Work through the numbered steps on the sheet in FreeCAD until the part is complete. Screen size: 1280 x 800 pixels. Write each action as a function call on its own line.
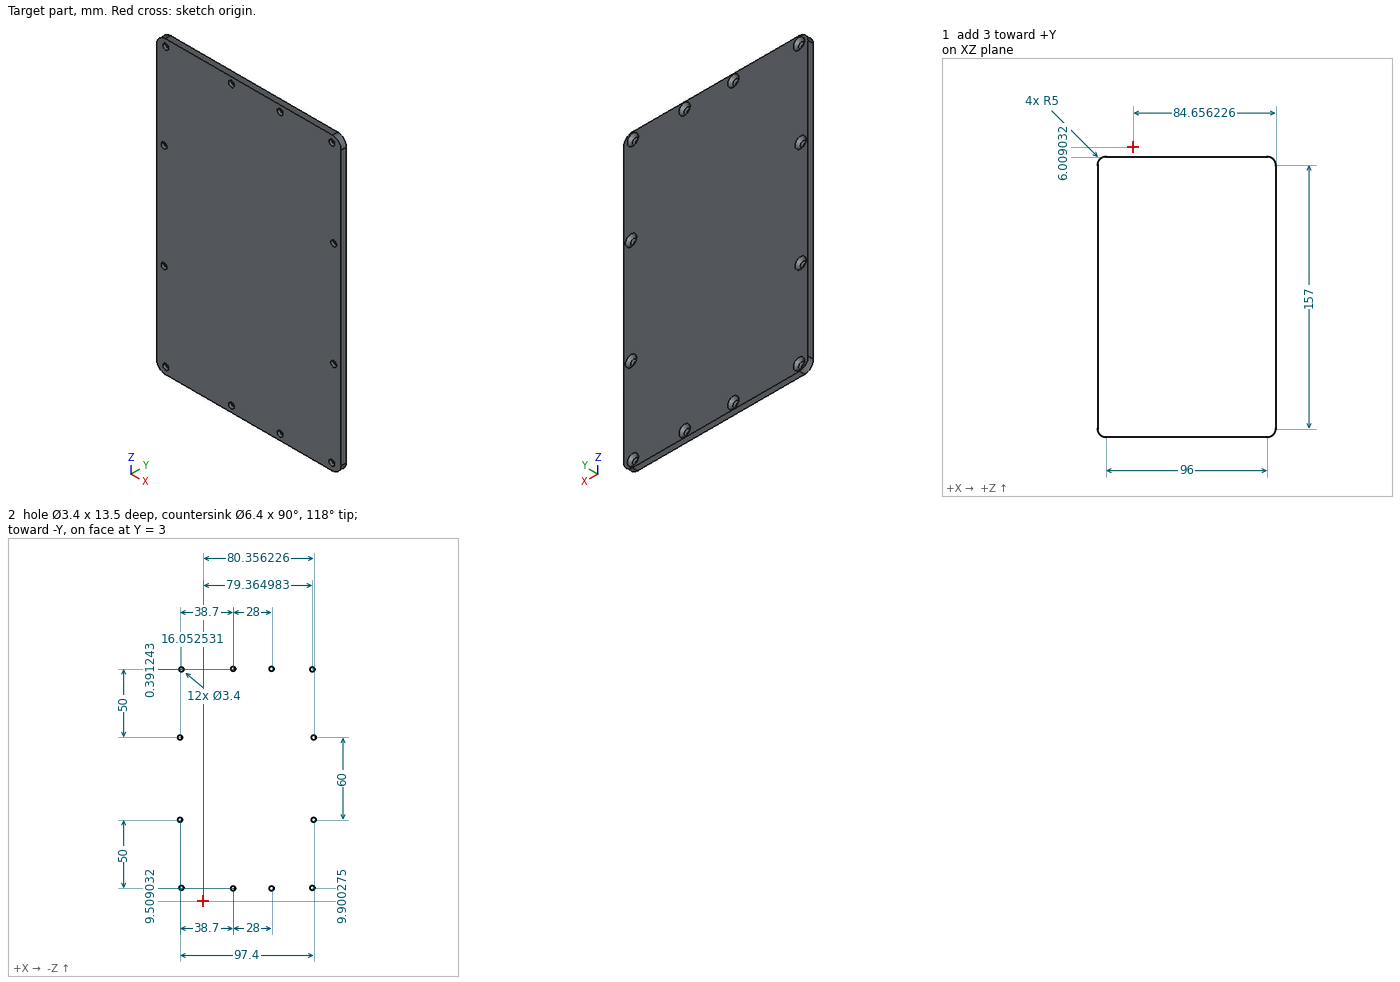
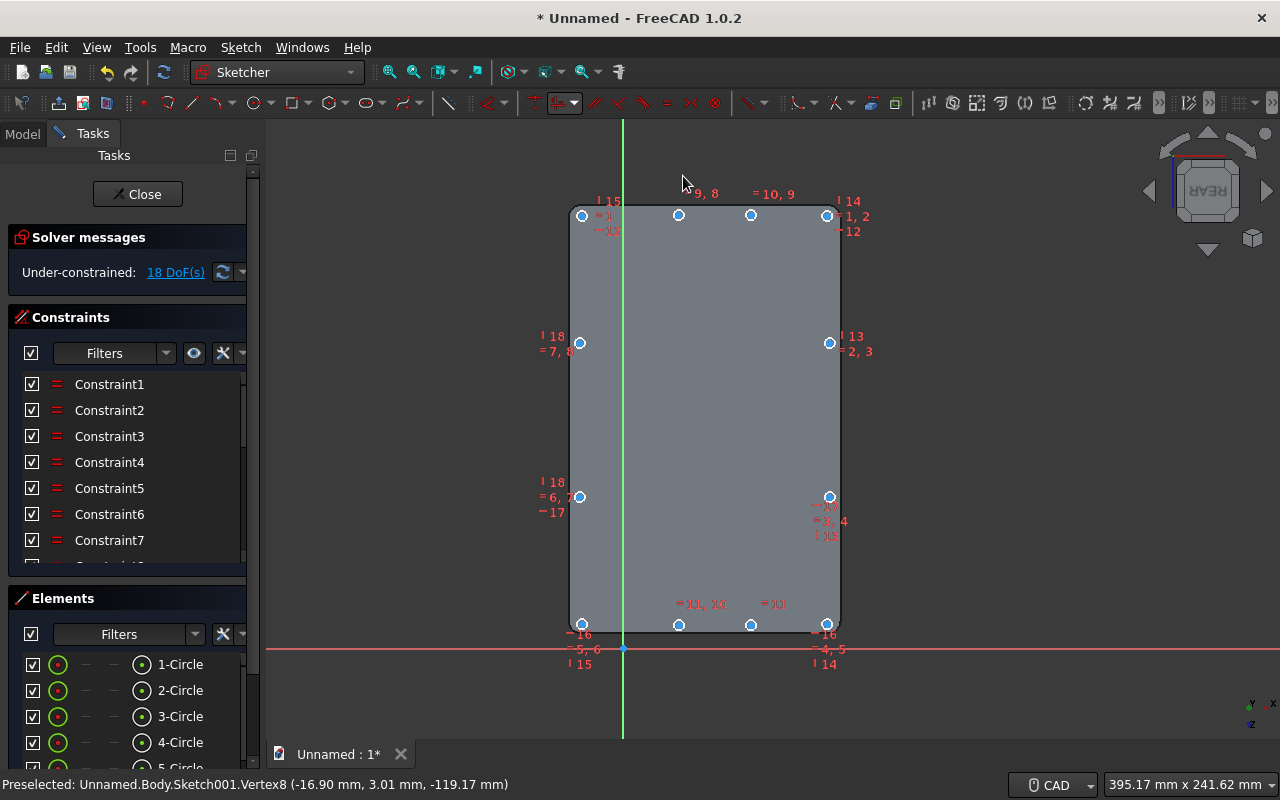
click(830, 343)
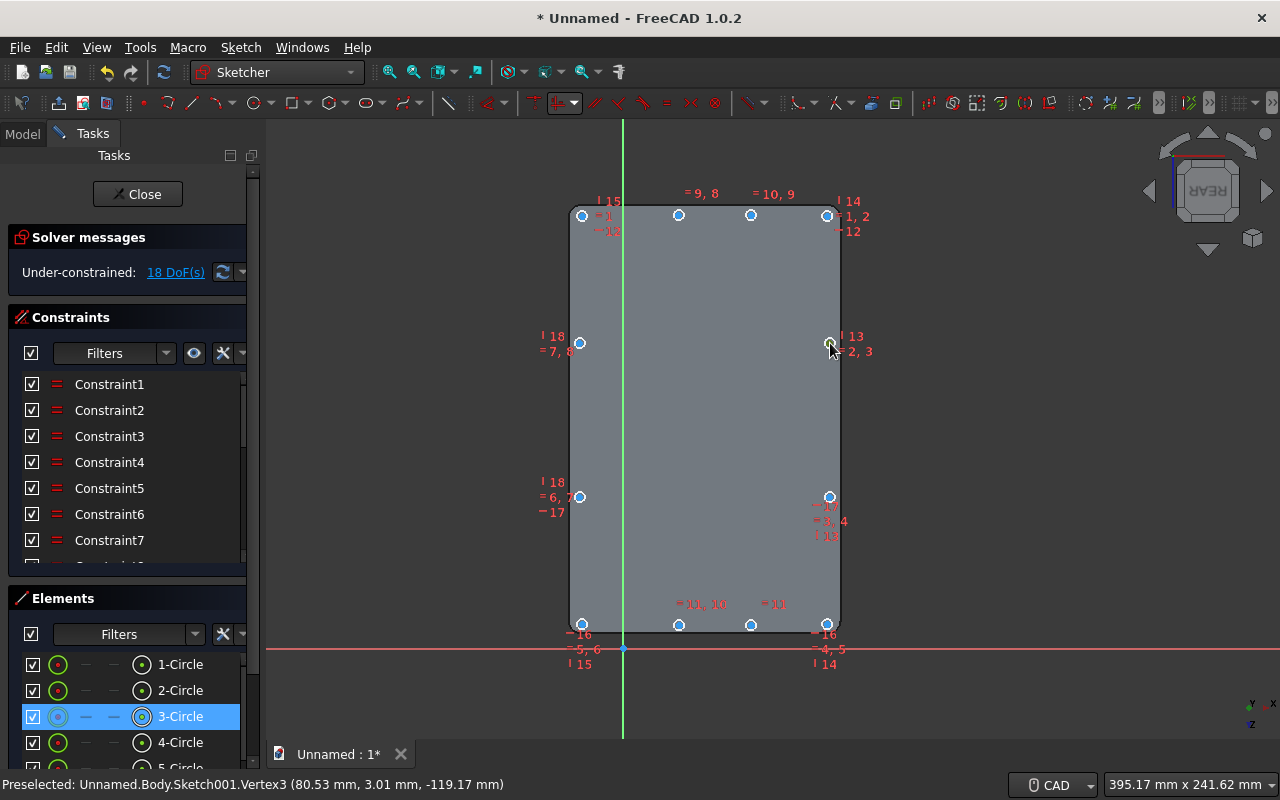
click(580, 343)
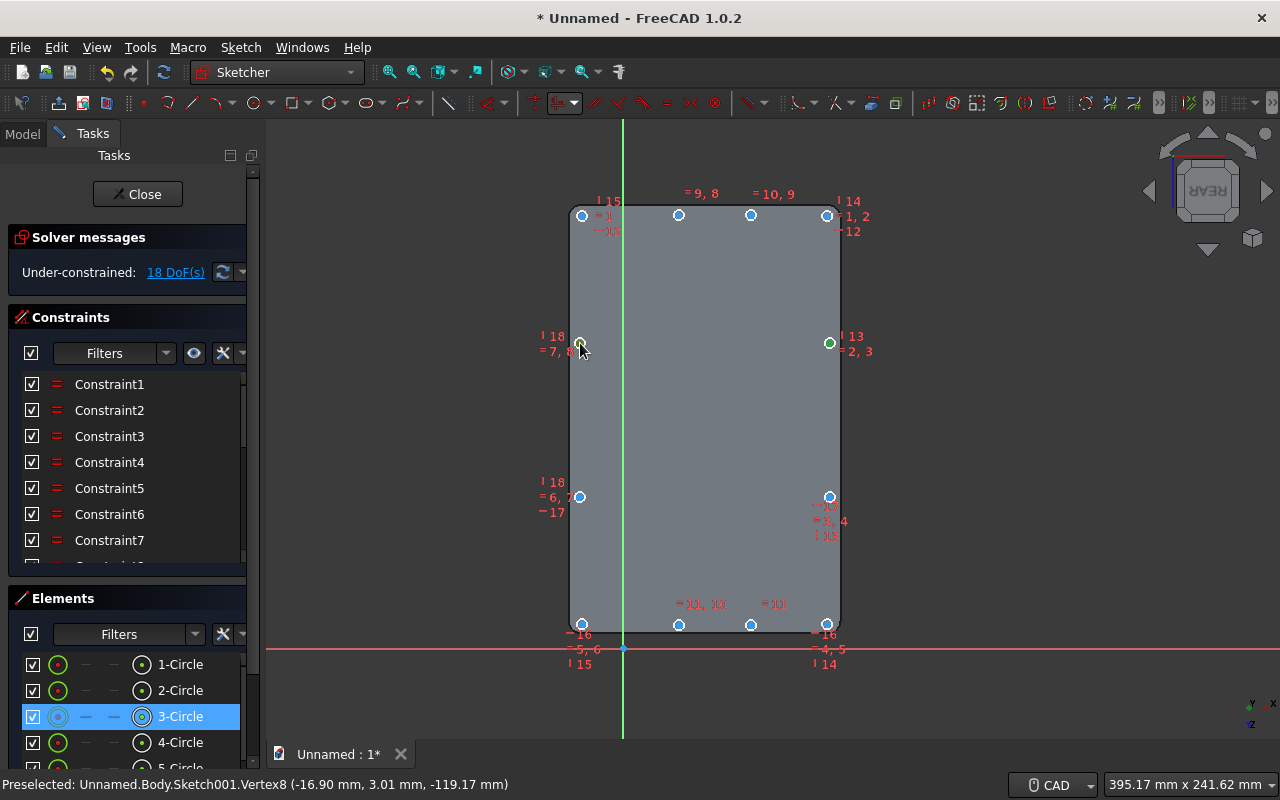
click(576, 104)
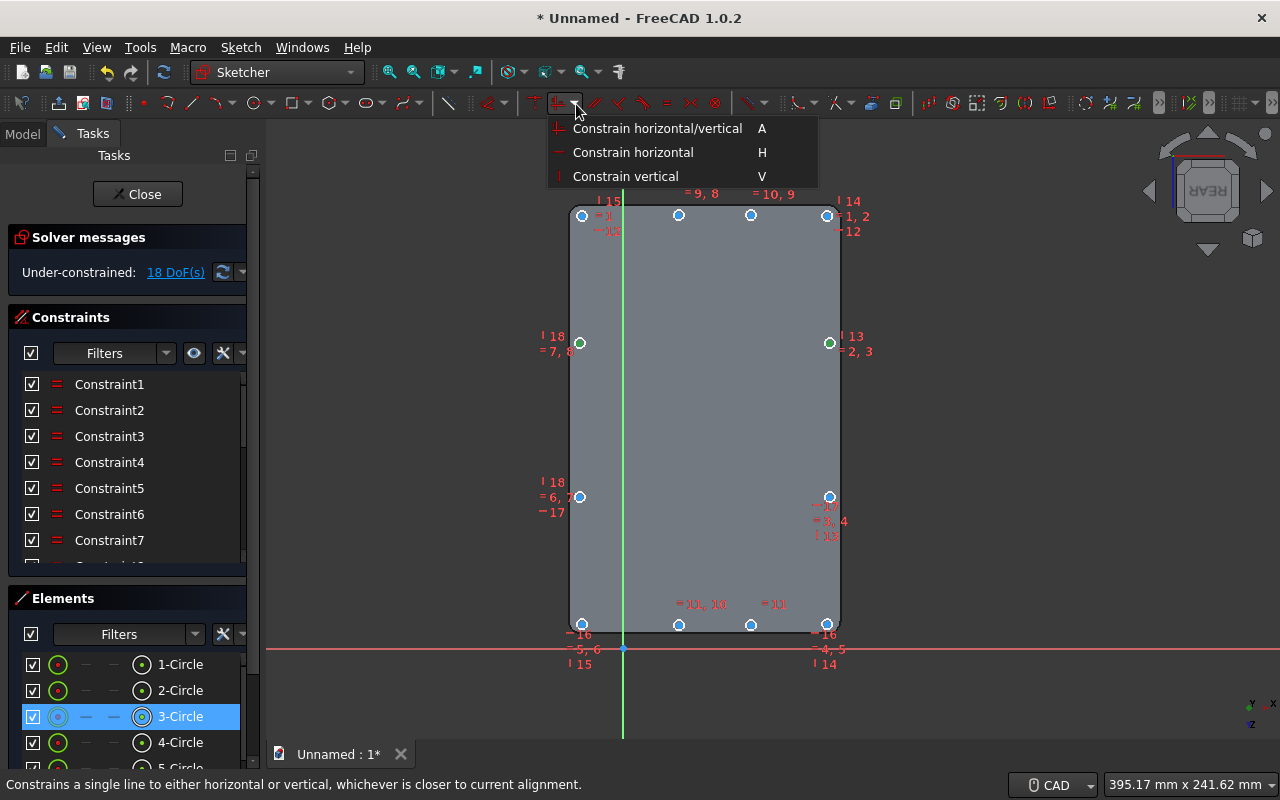
click(683, 152)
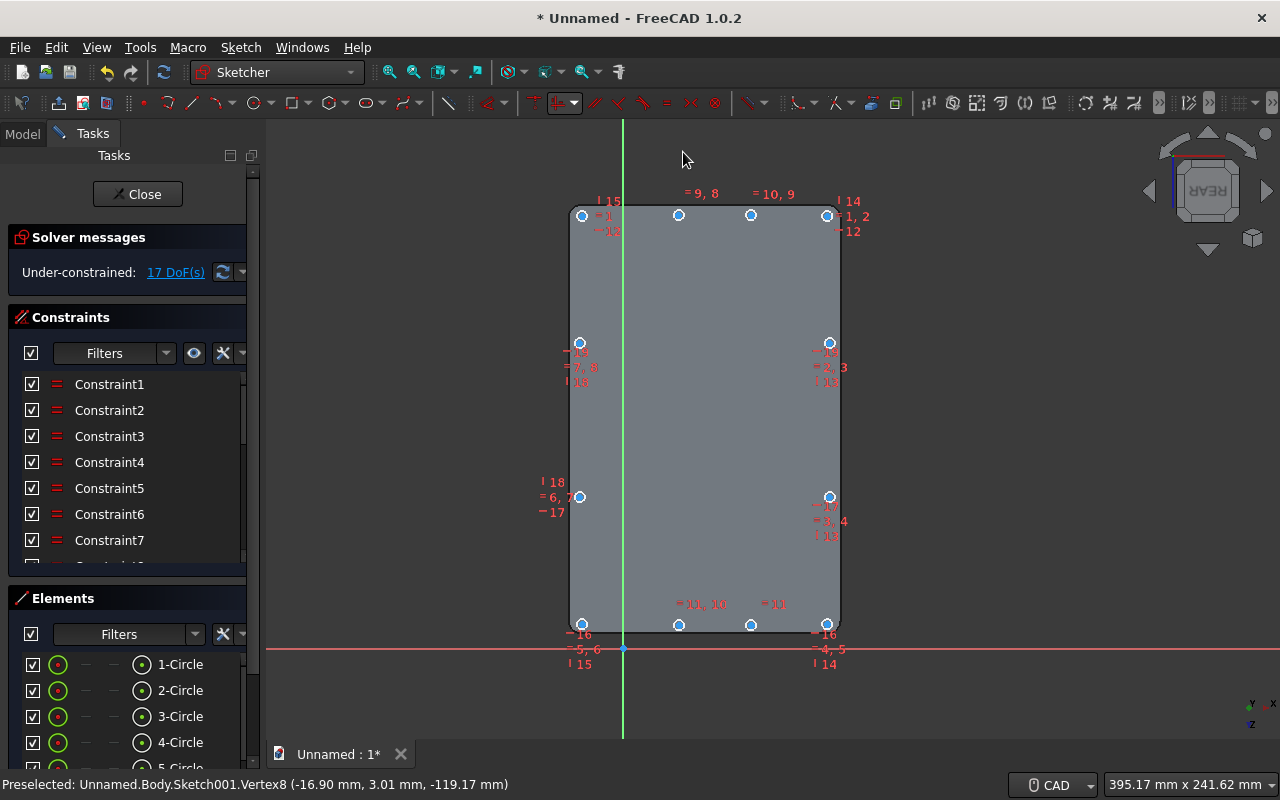
click(679, 215)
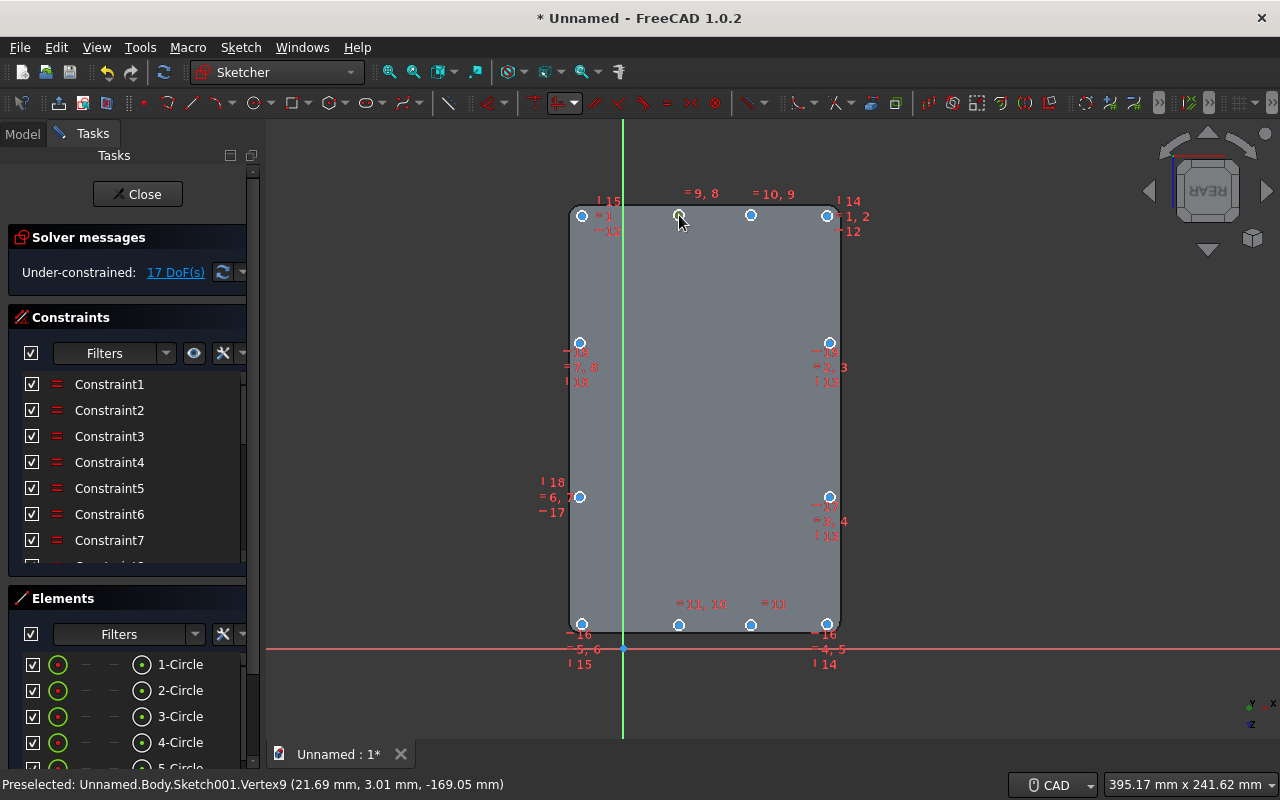
click(751, 215)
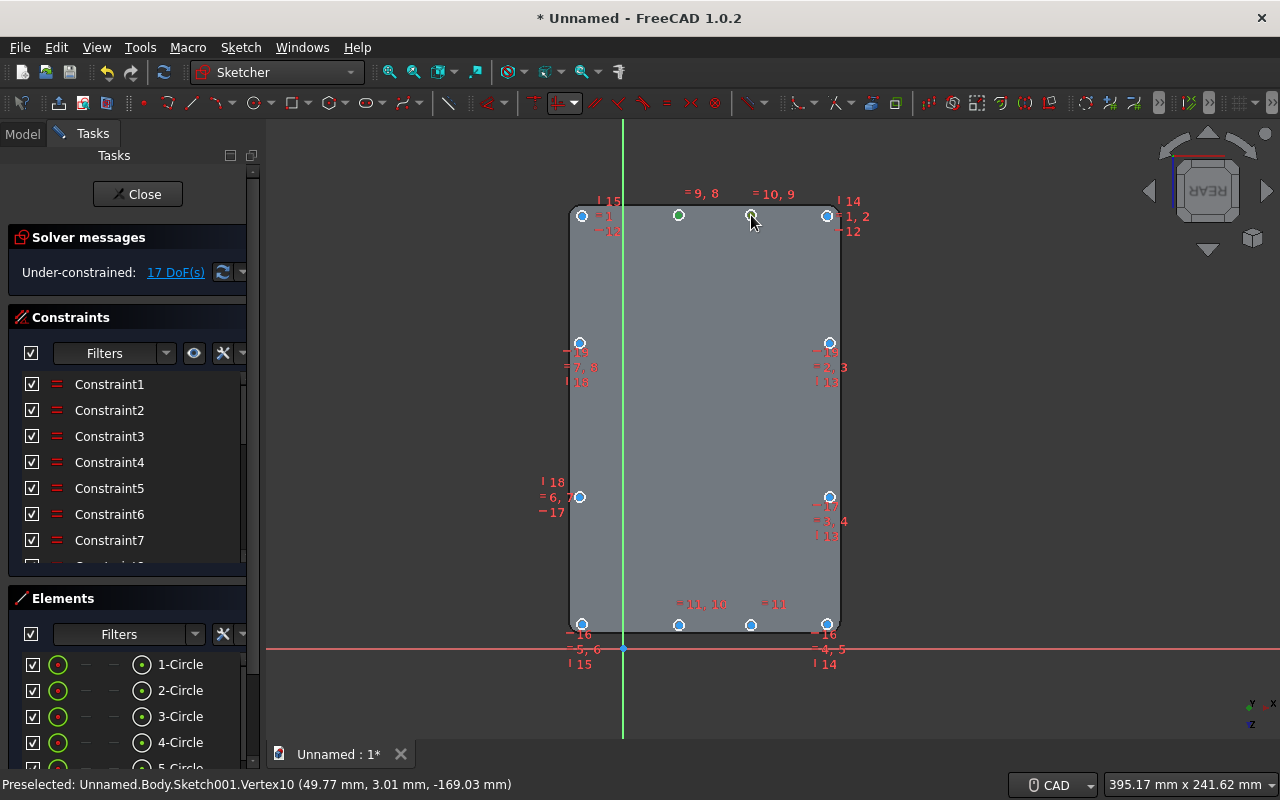
click(576, 104)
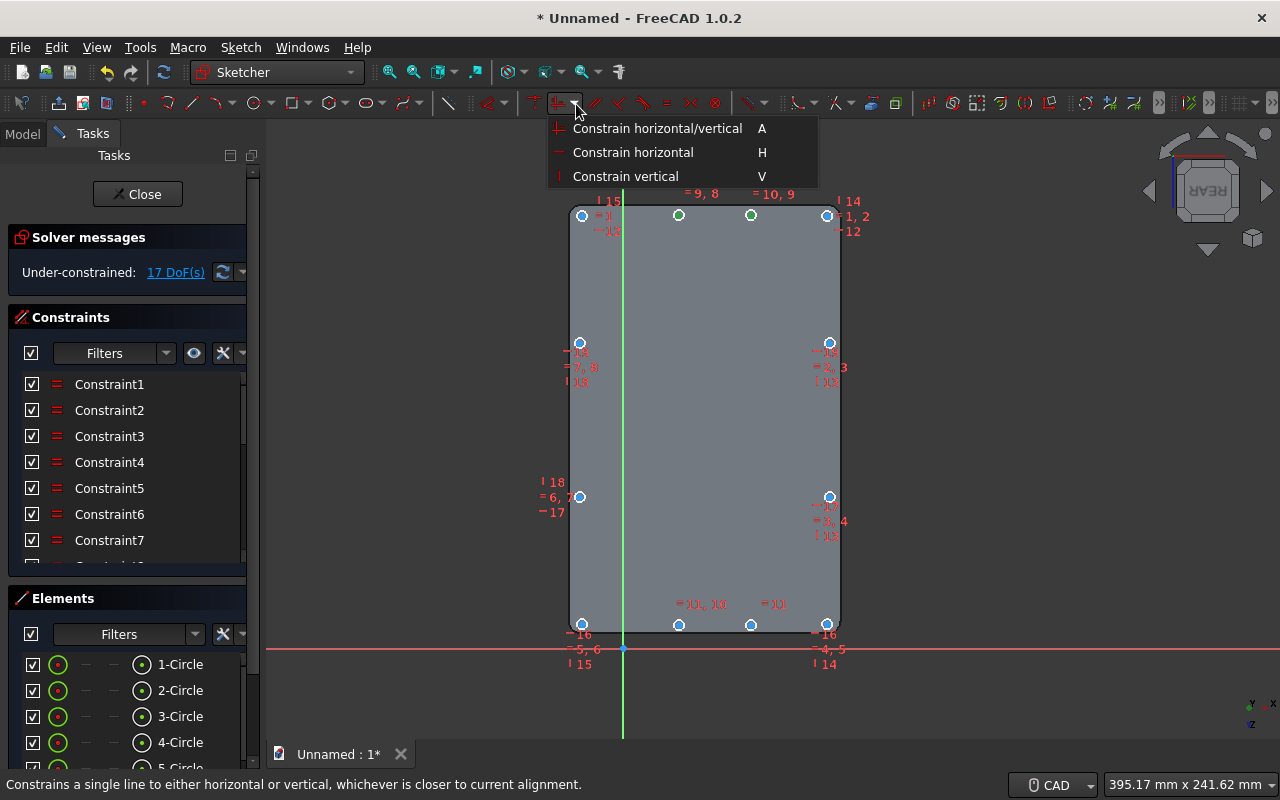
click(683, 152)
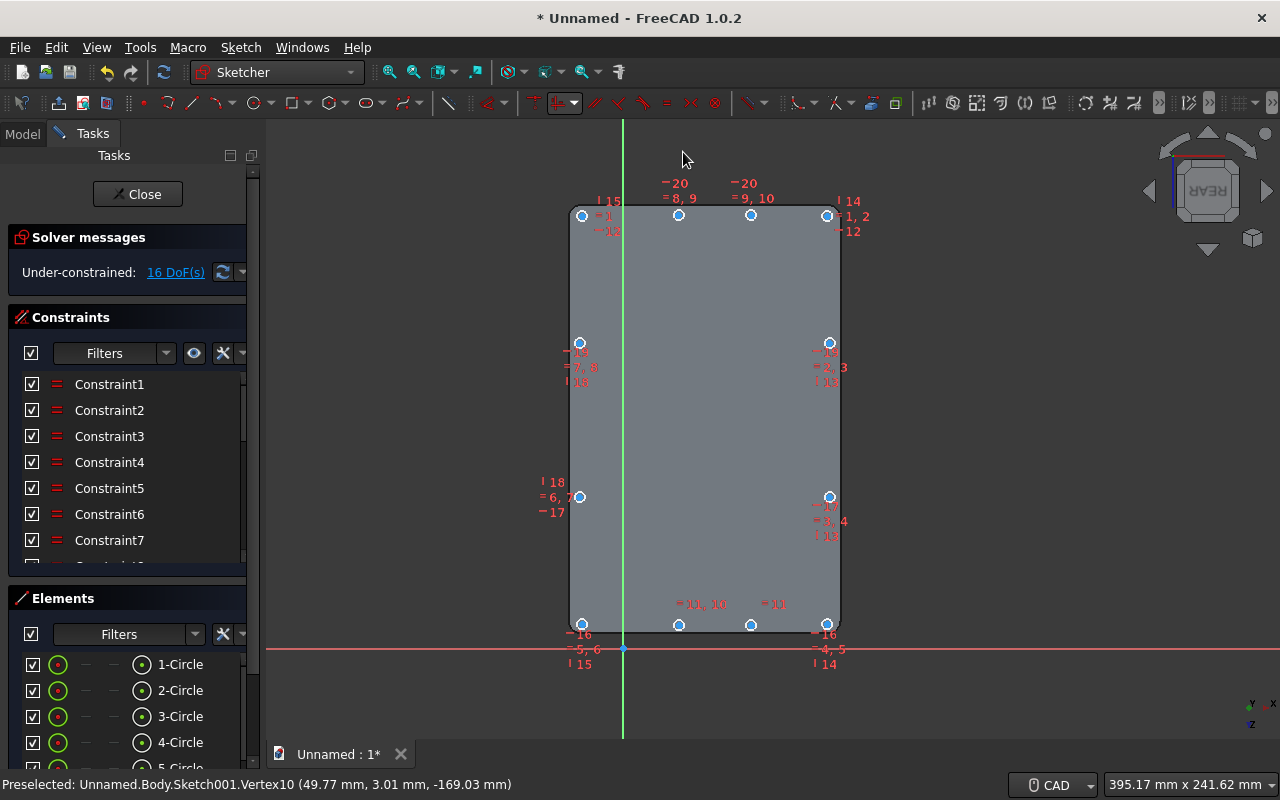
click(679, 625)